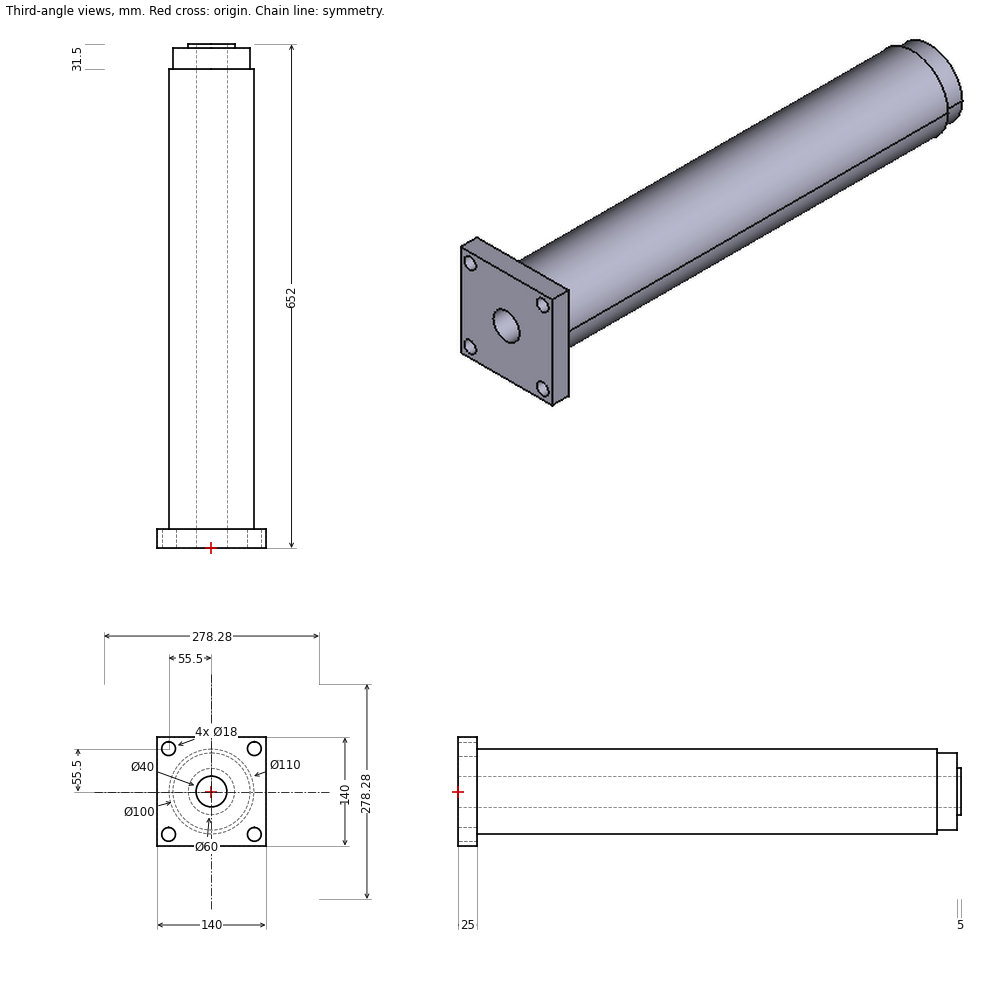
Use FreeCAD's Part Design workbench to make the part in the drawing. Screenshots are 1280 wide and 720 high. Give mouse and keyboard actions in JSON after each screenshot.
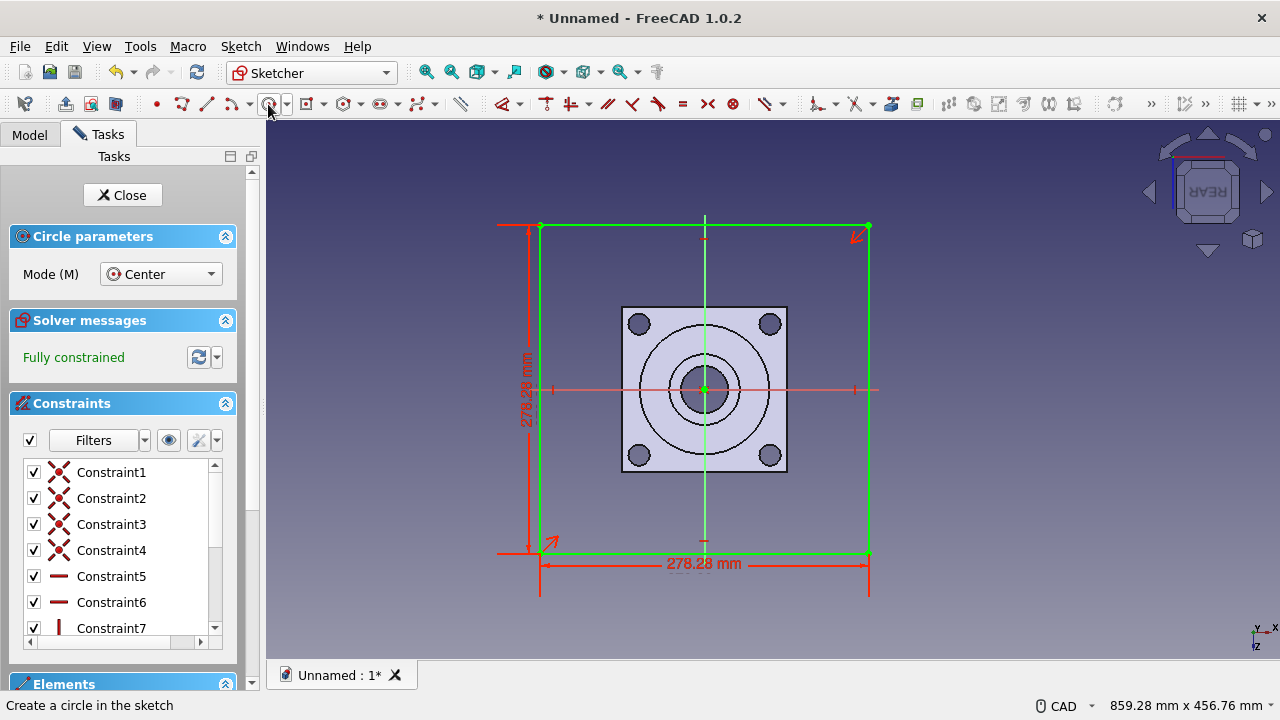
{"action": "left_click", "coordinate": [705, 390]}
{"action": "mouse_move", "coordinate": [746, 348]}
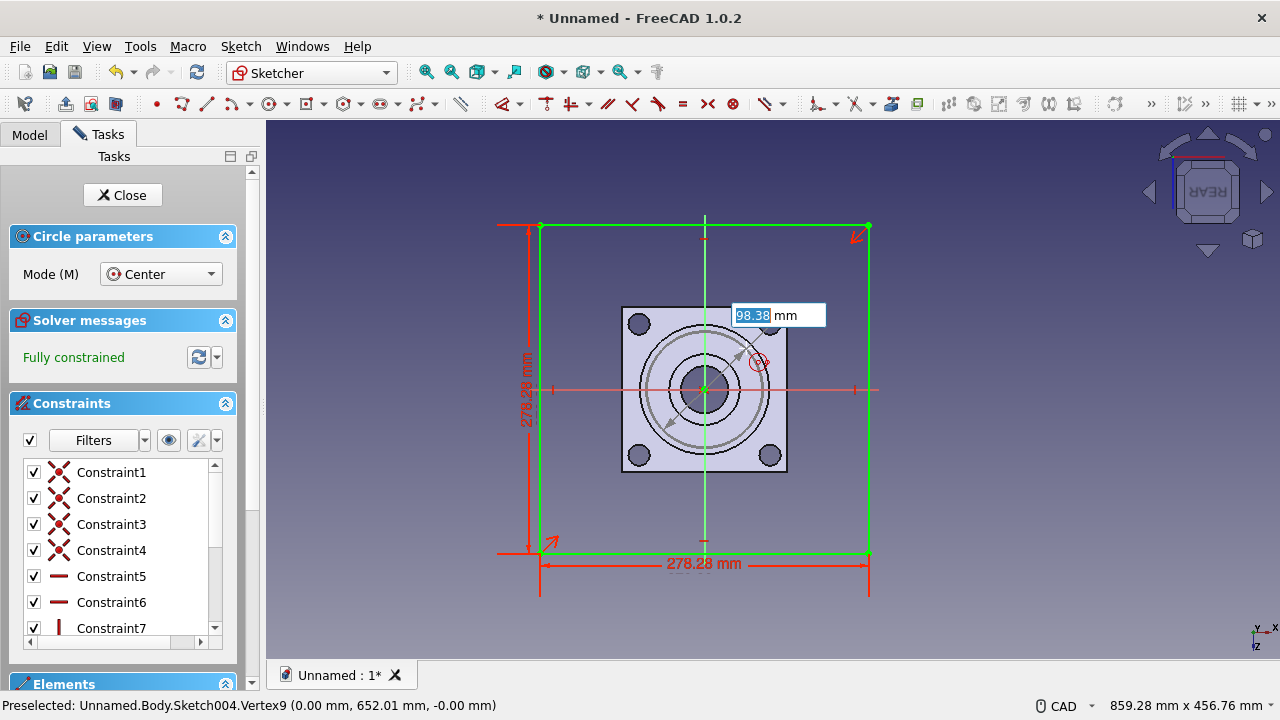
{"action": "type", "text": "100"}
{"action": "key", "text": "Return"}
{"action": "key", "text": "Escape"}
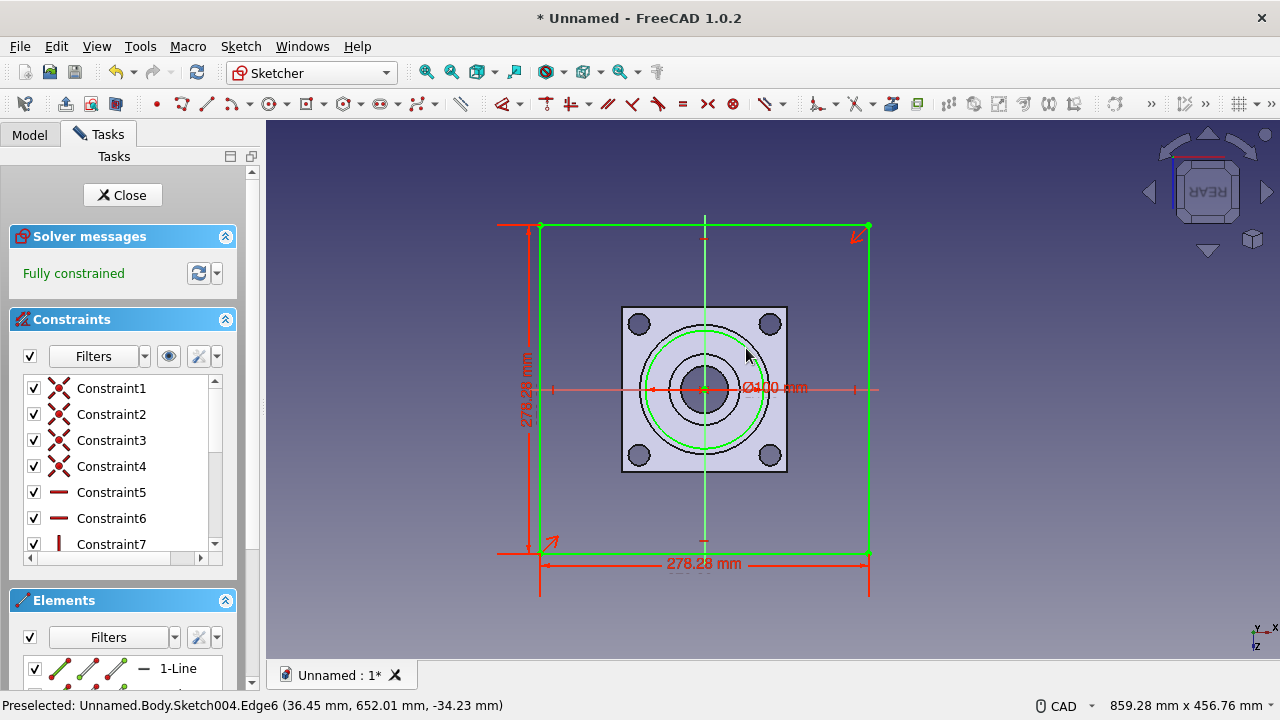
{"action": "left_click", "coordinate": [123, 195]}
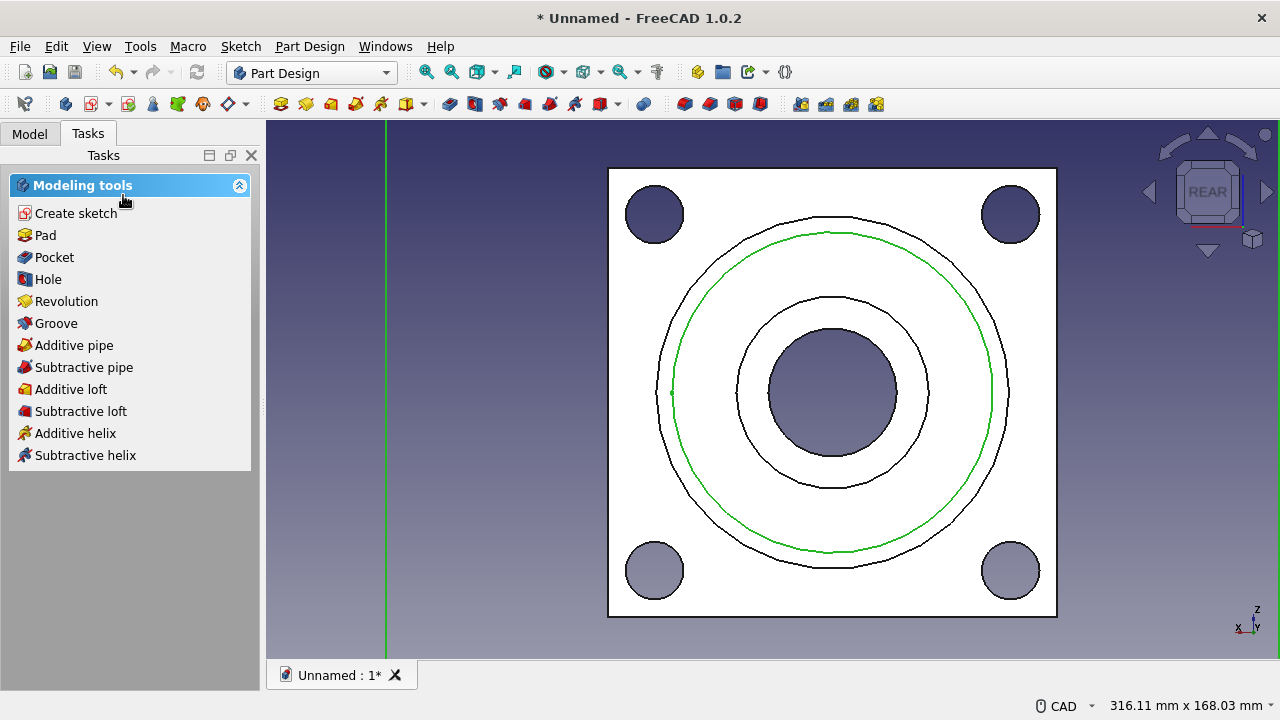
{"action": "left_click", "coordinate": [450, 104]}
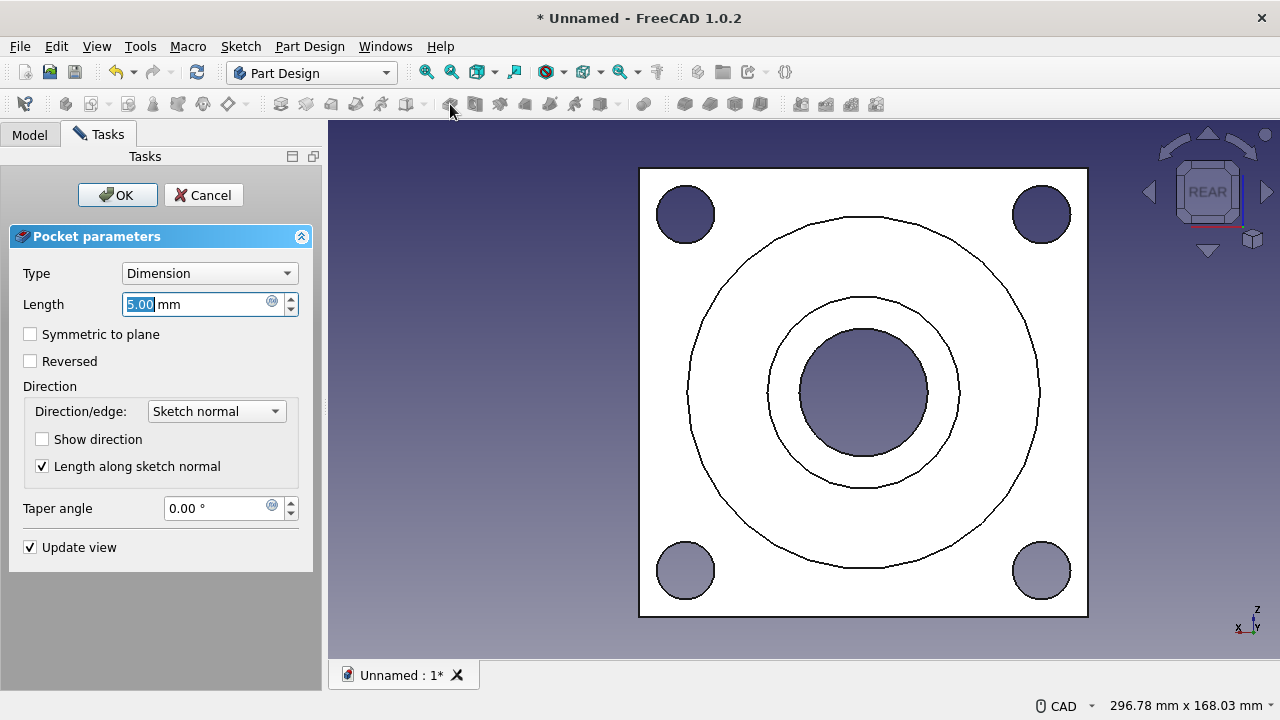
{"action": "type", "text": "31.5"}
{"action": "key", "text": "Tab"}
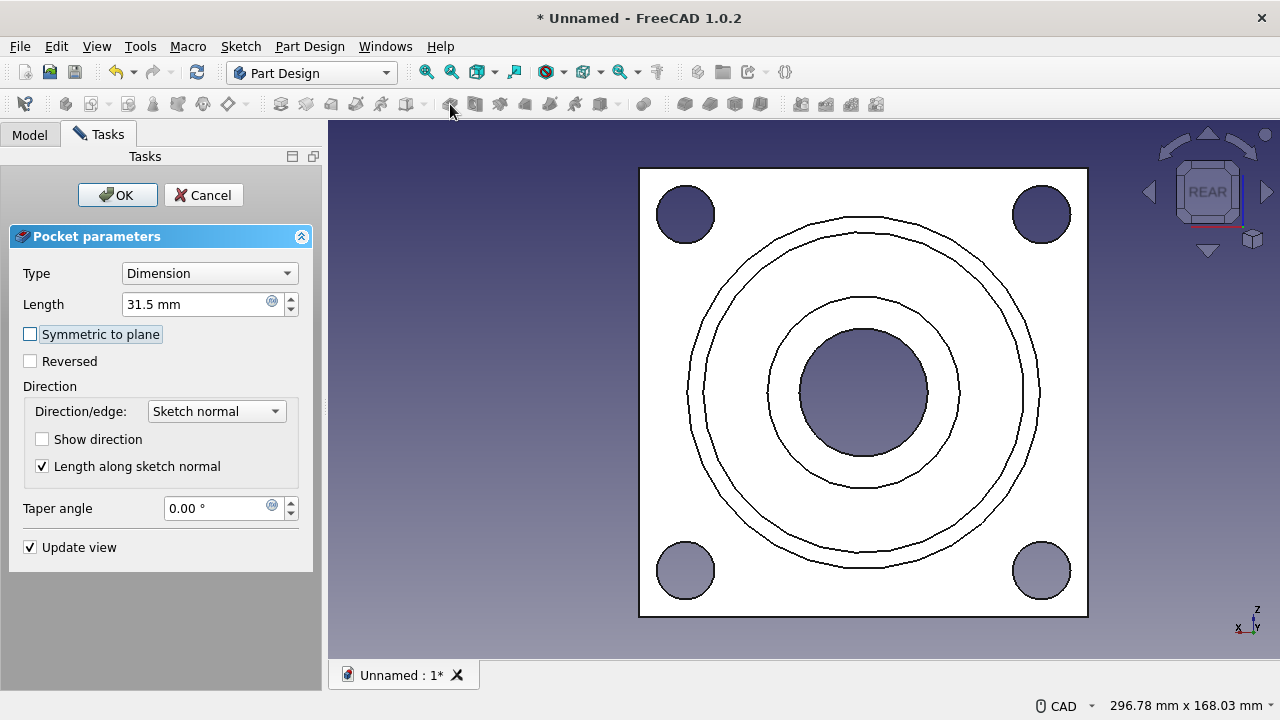
{"action": "left_click", "coordinate": [118, 195]}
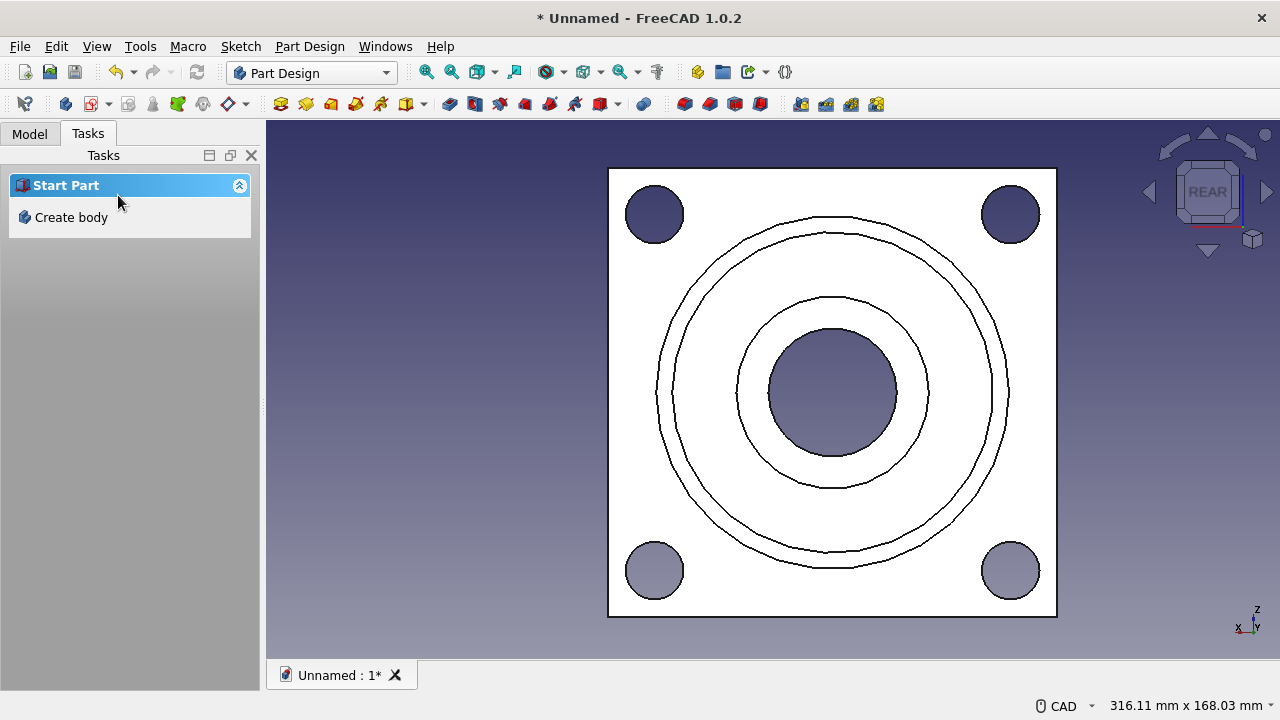
{"action": "key", "text": "0"}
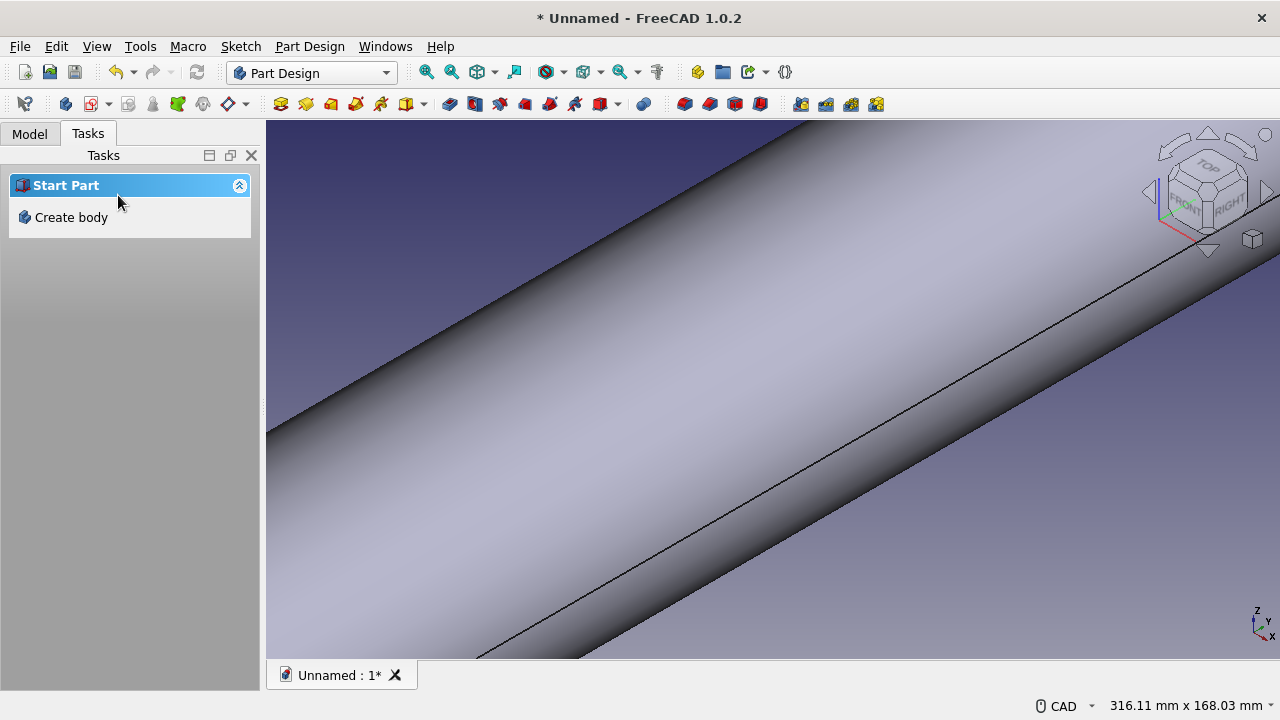
{"action": "left_click", "coordinate": [427, 72]}